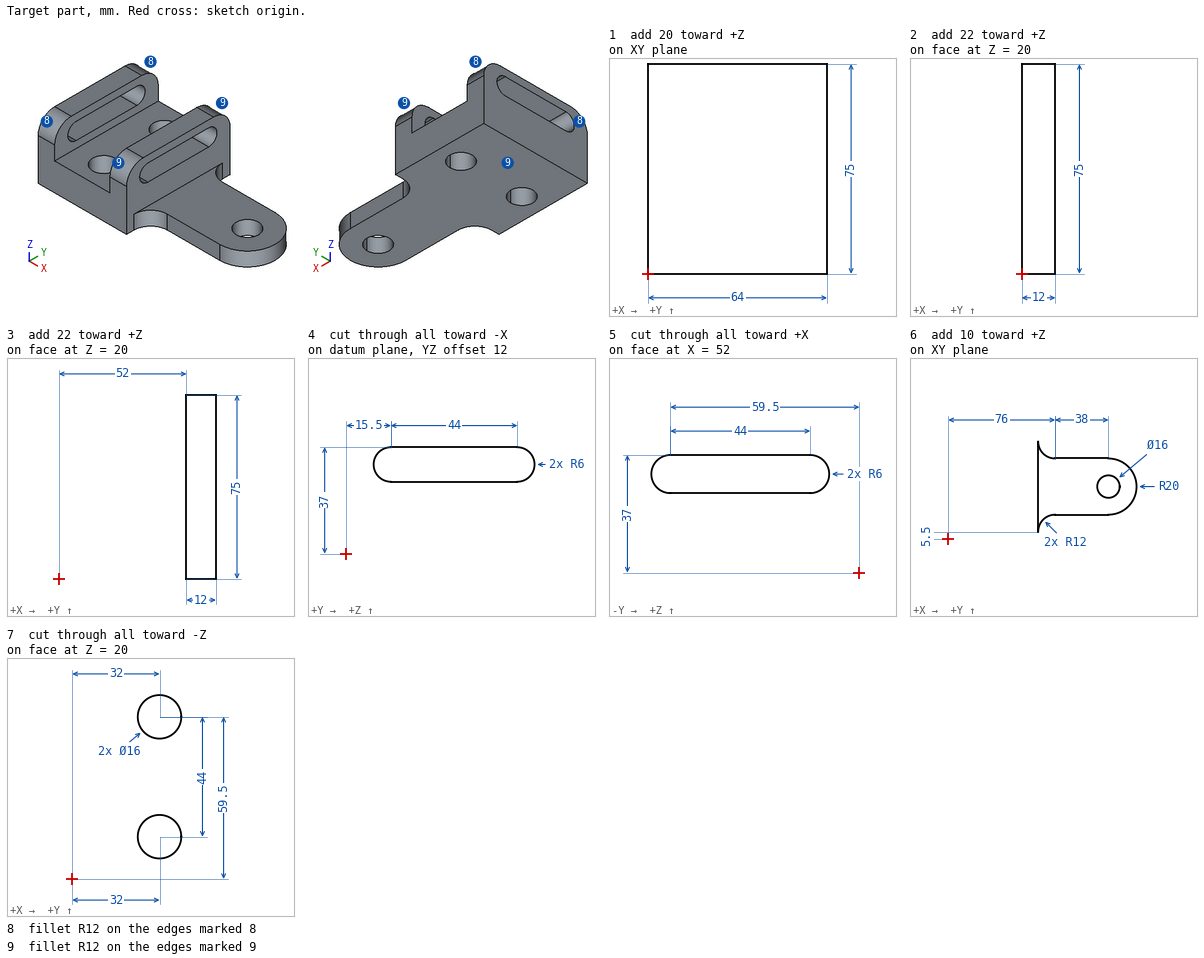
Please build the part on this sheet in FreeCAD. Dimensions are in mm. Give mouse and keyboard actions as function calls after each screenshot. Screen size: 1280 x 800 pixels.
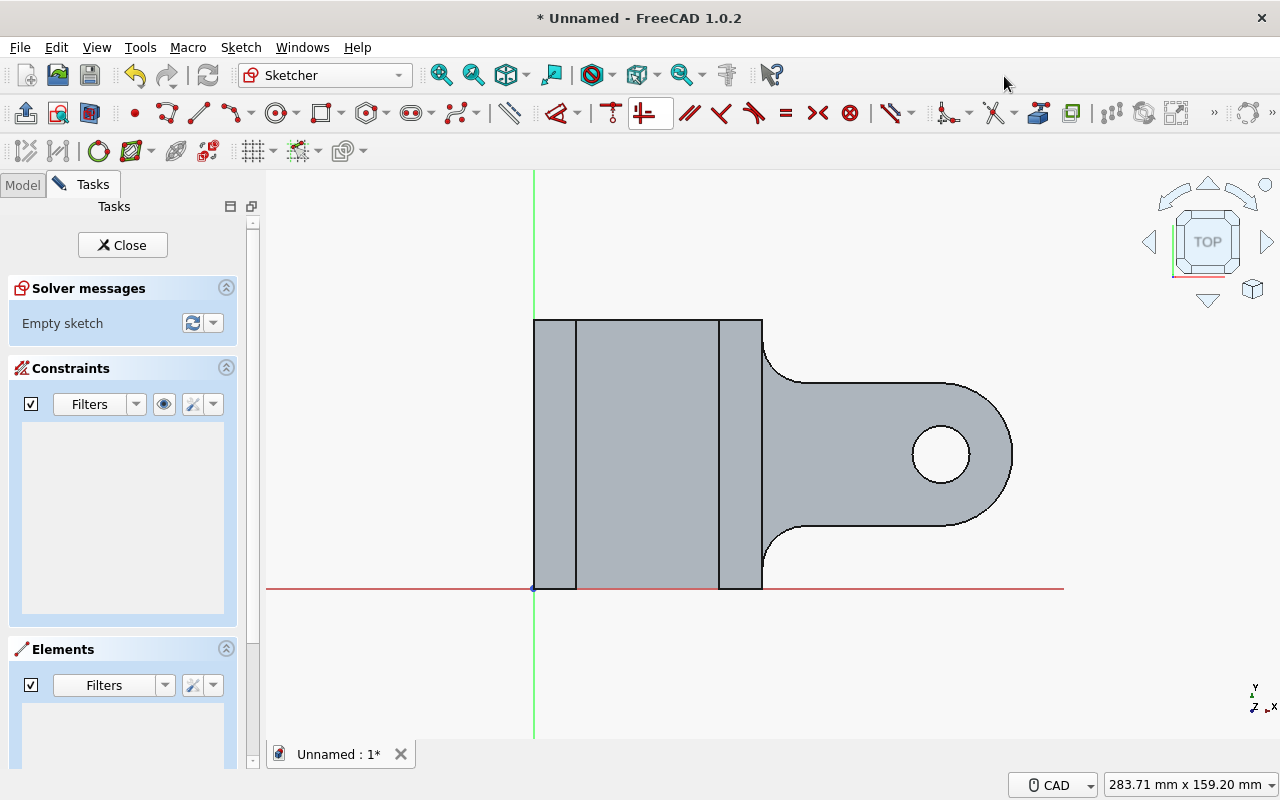
scroll(403, 495, up, 2)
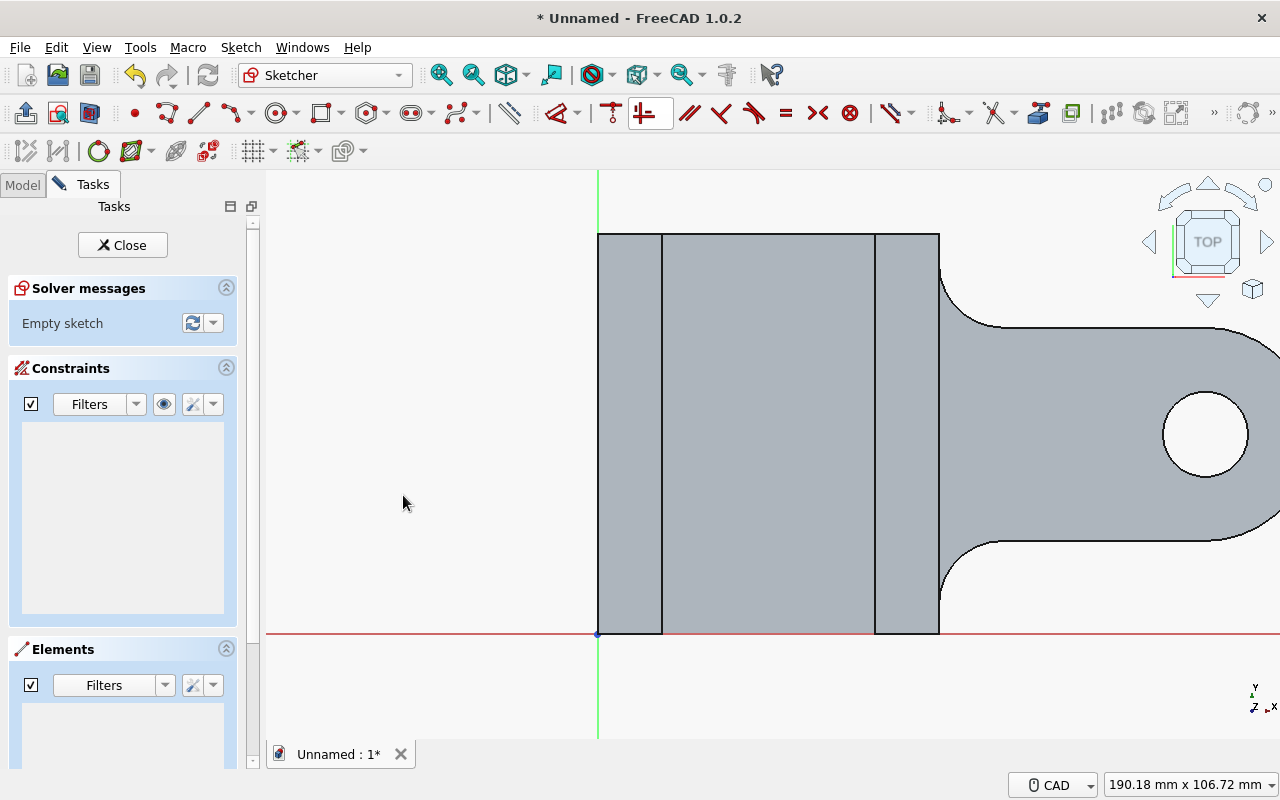
click(276, 114)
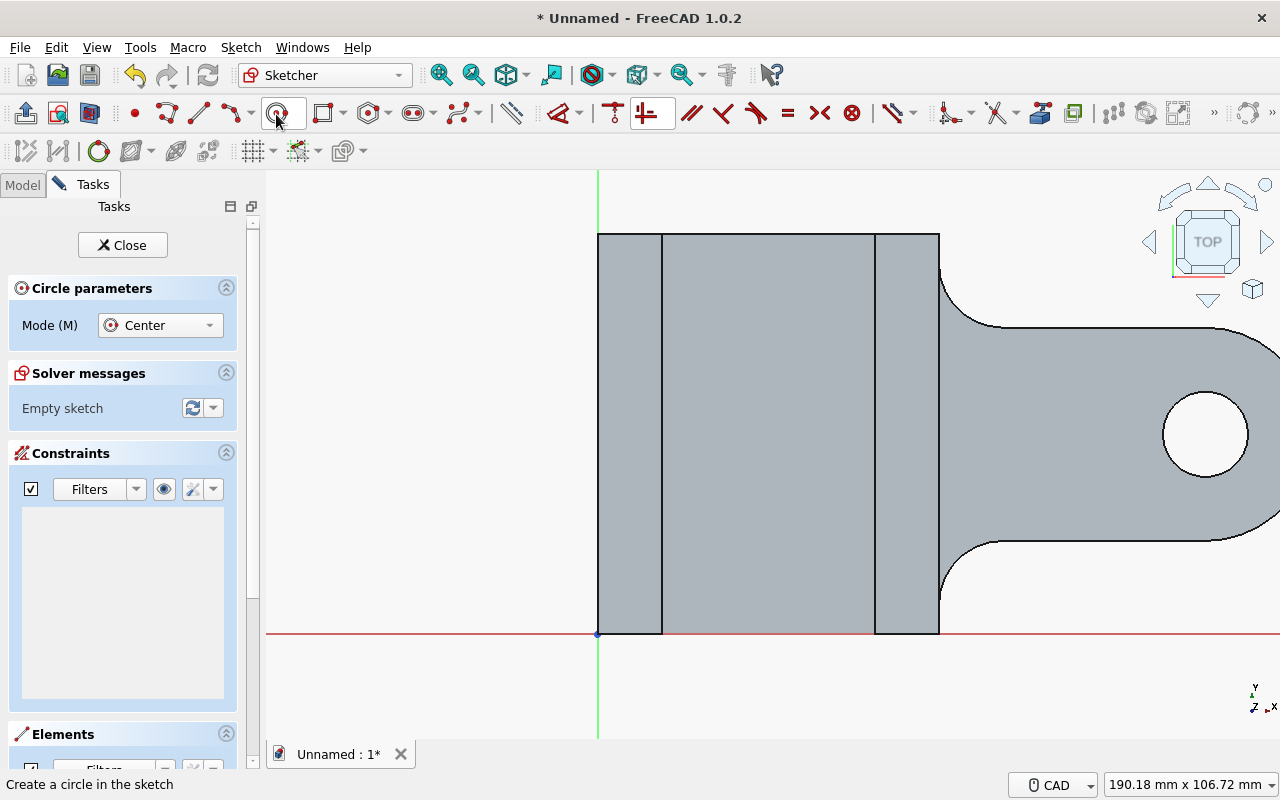
click(768, 317)
click(798, 287)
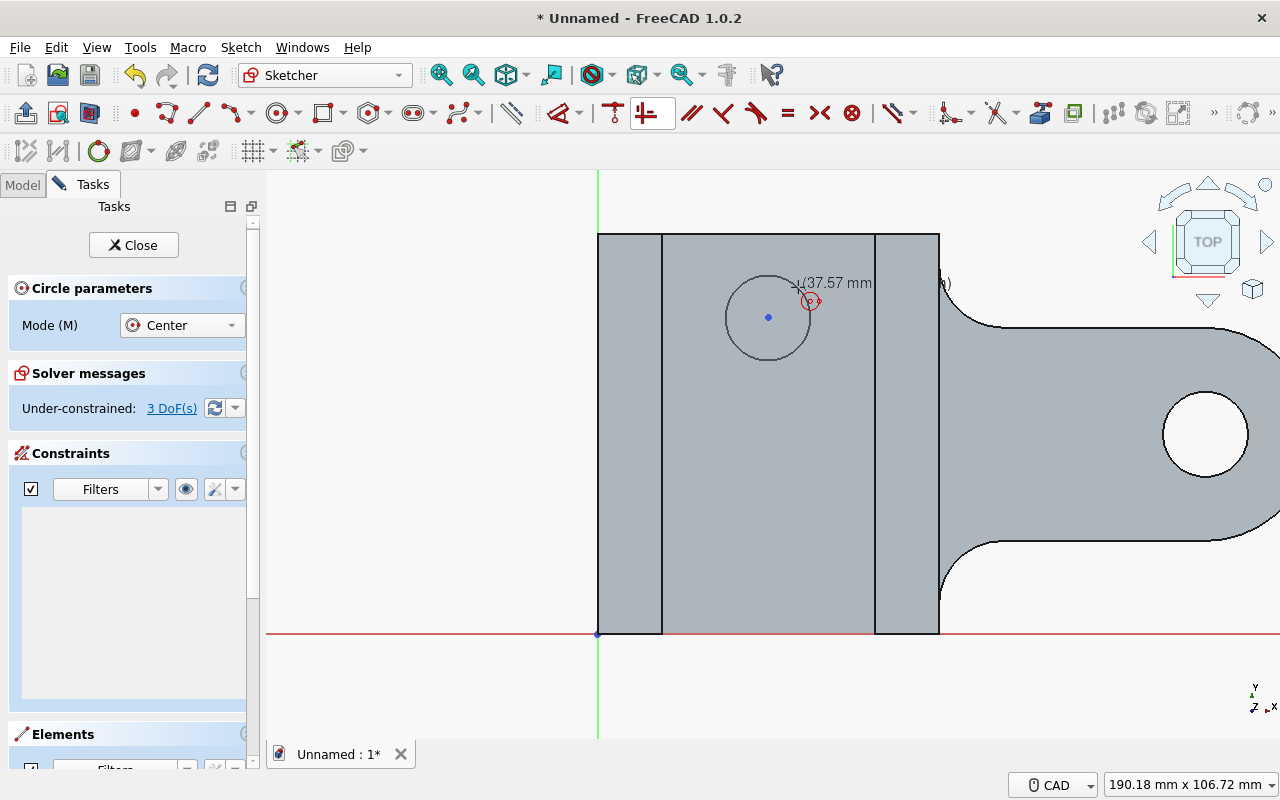
click(768, 552)
click(798, 521)
key(Escape)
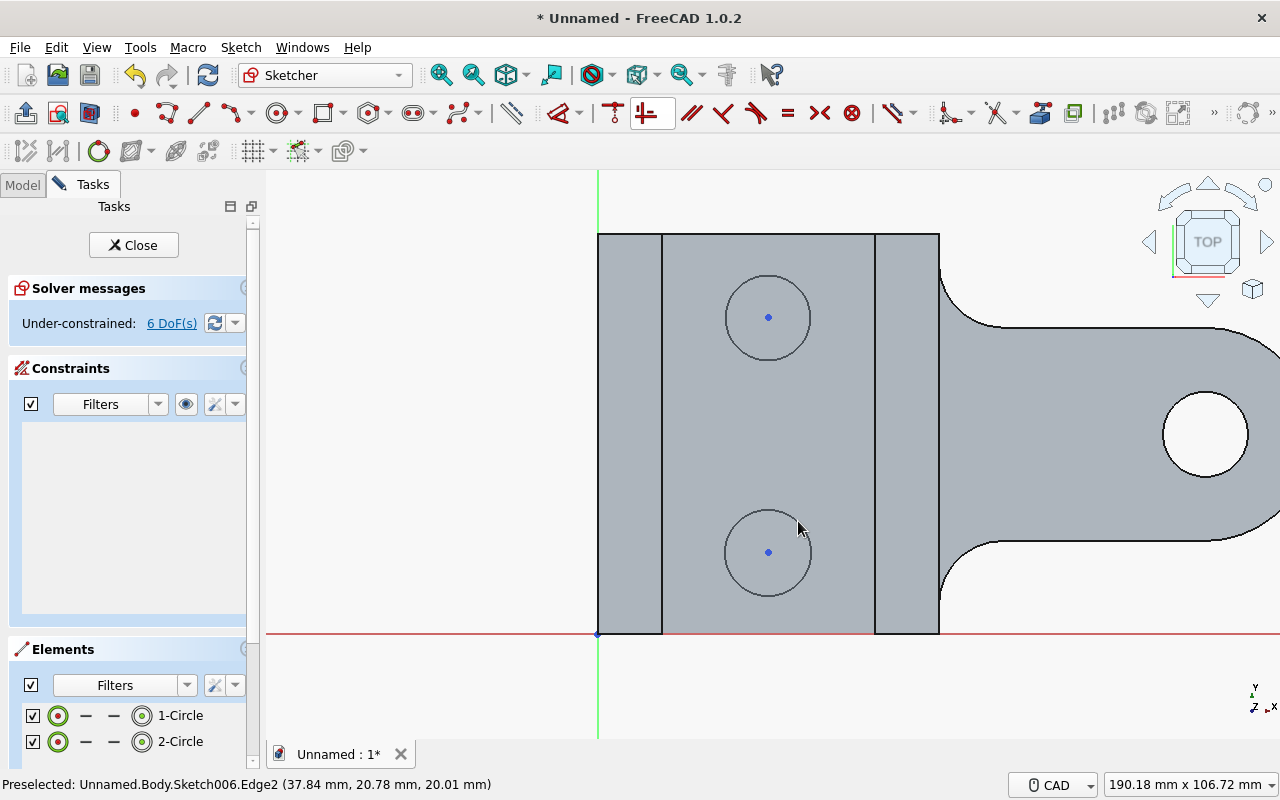
click(798, 288)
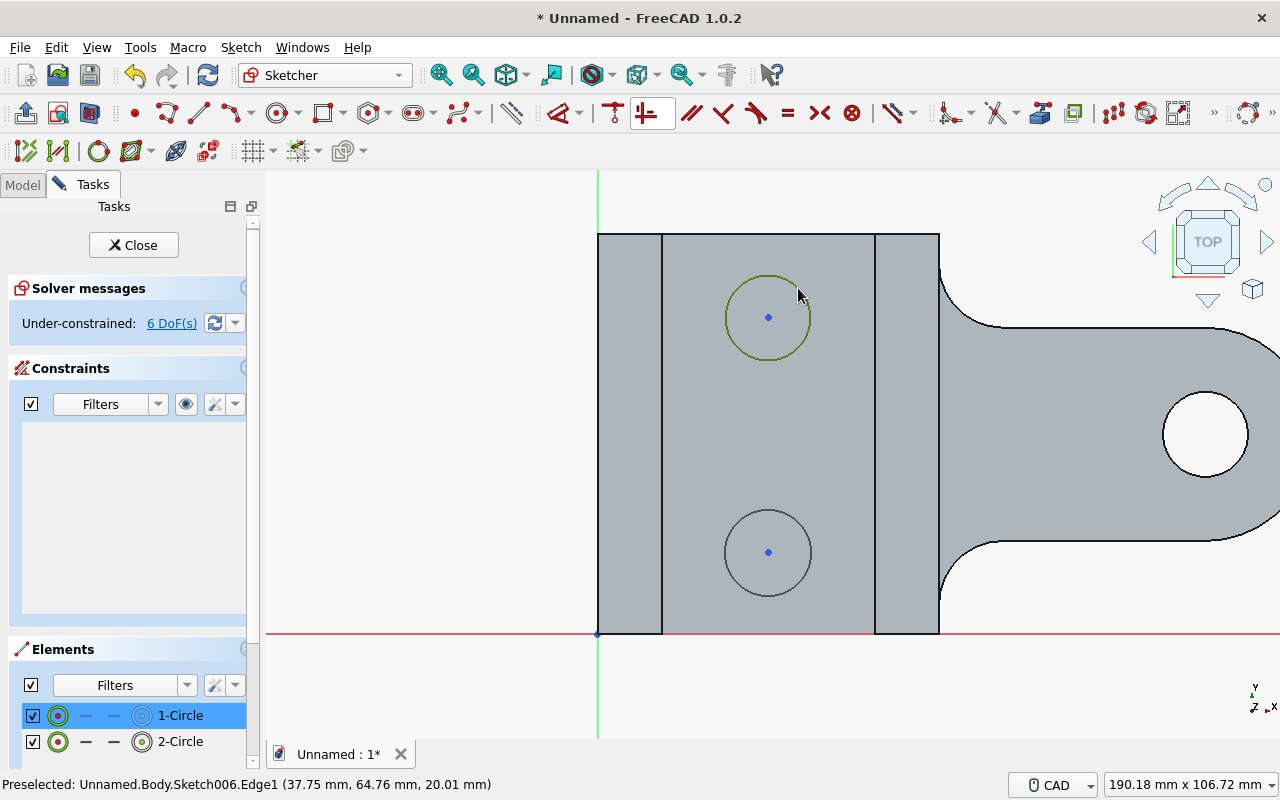
click(798, 522)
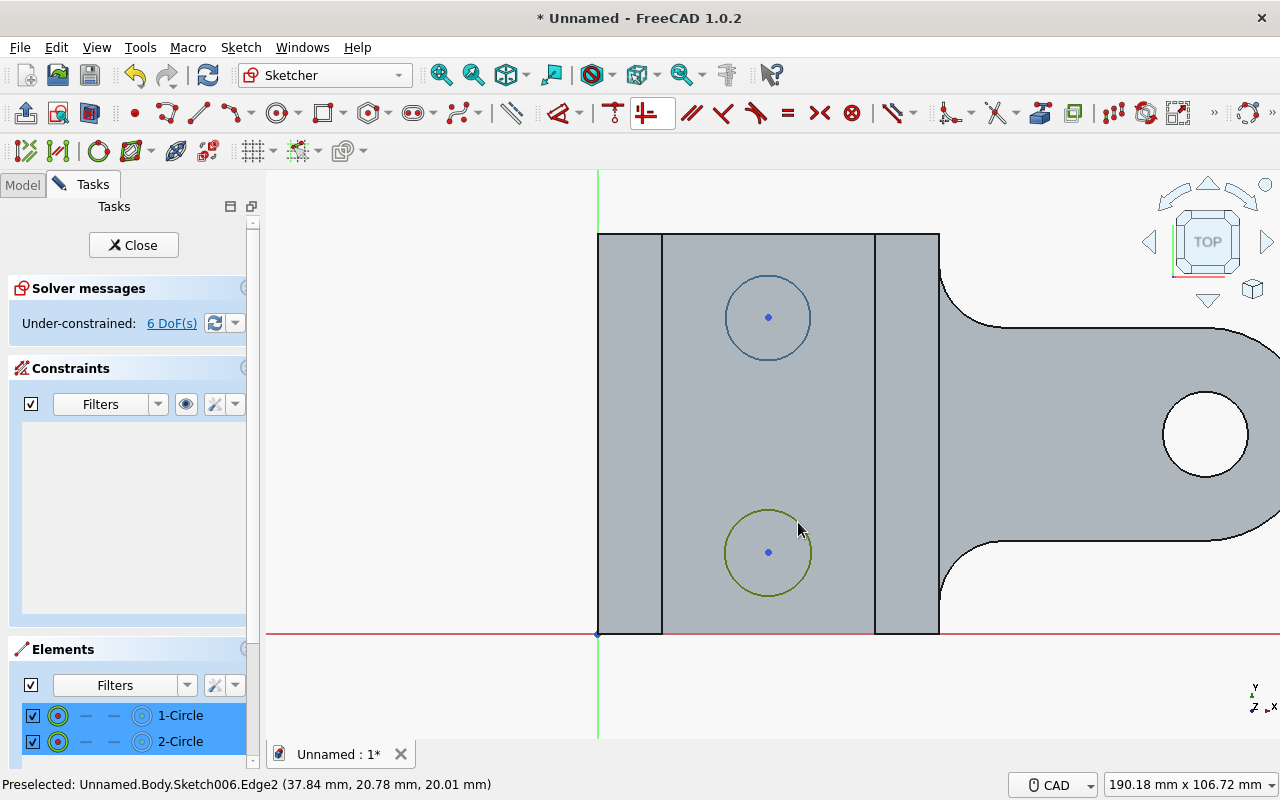
click(788, 114)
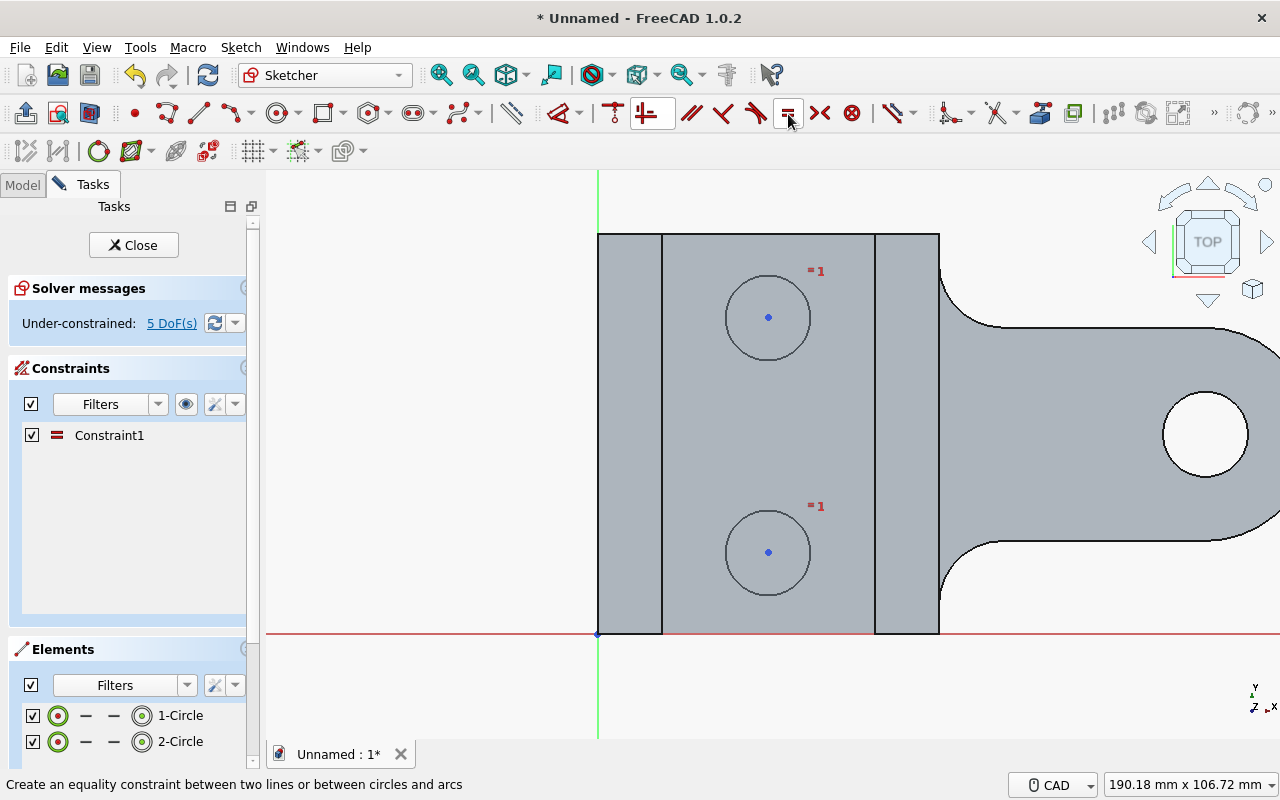
click(558, 114)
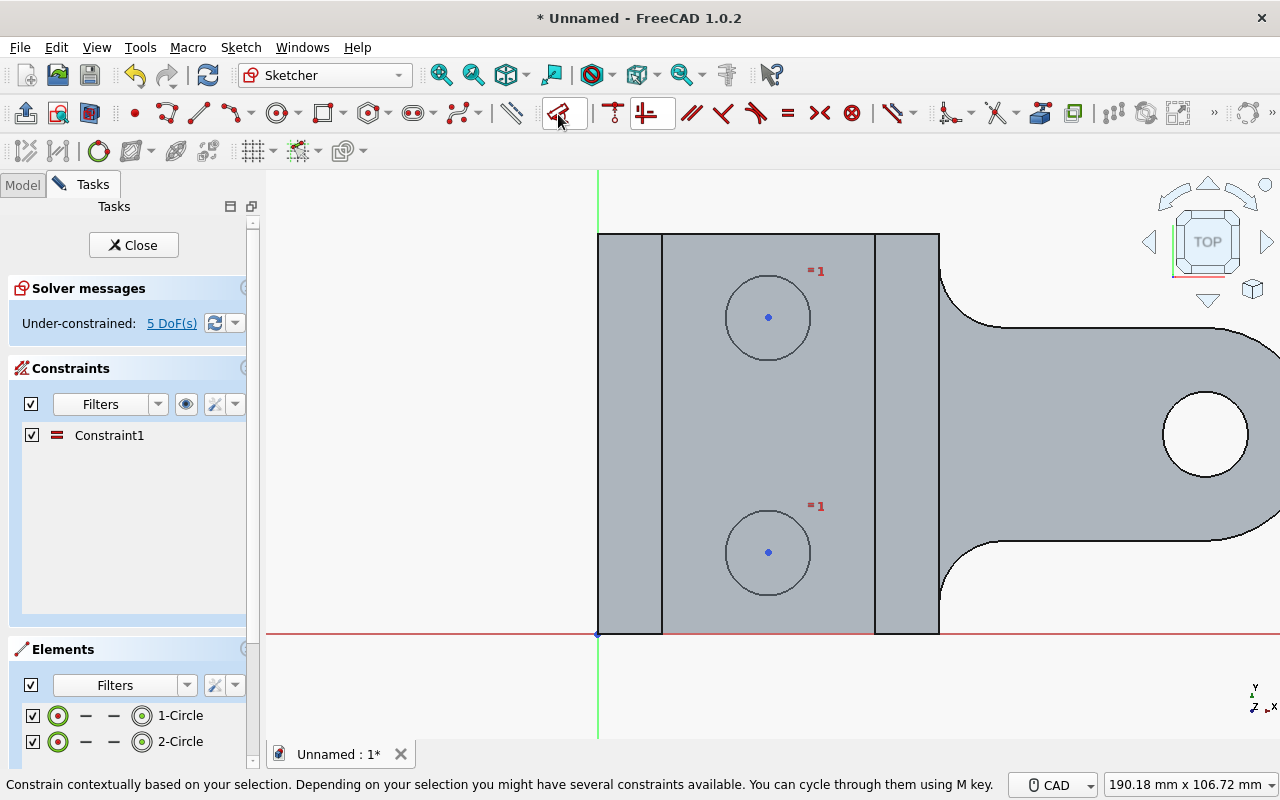
click(798, 288)
click(821, 265)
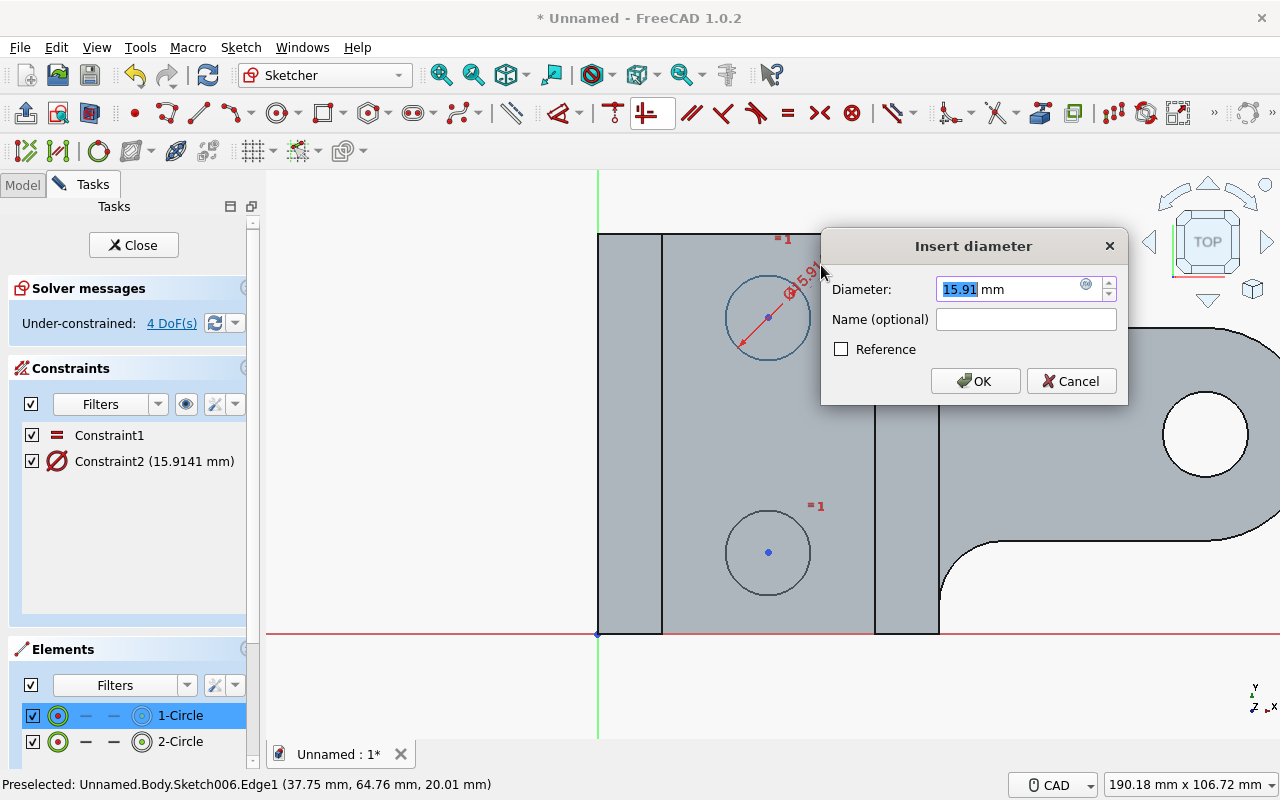
text(16)
key(Return)